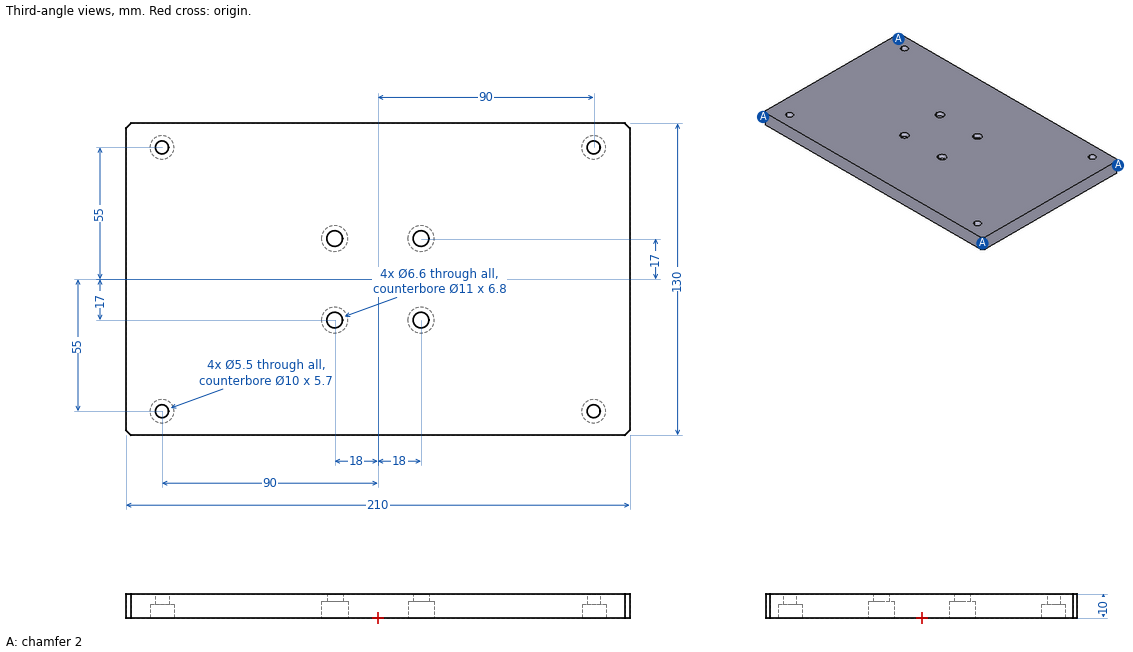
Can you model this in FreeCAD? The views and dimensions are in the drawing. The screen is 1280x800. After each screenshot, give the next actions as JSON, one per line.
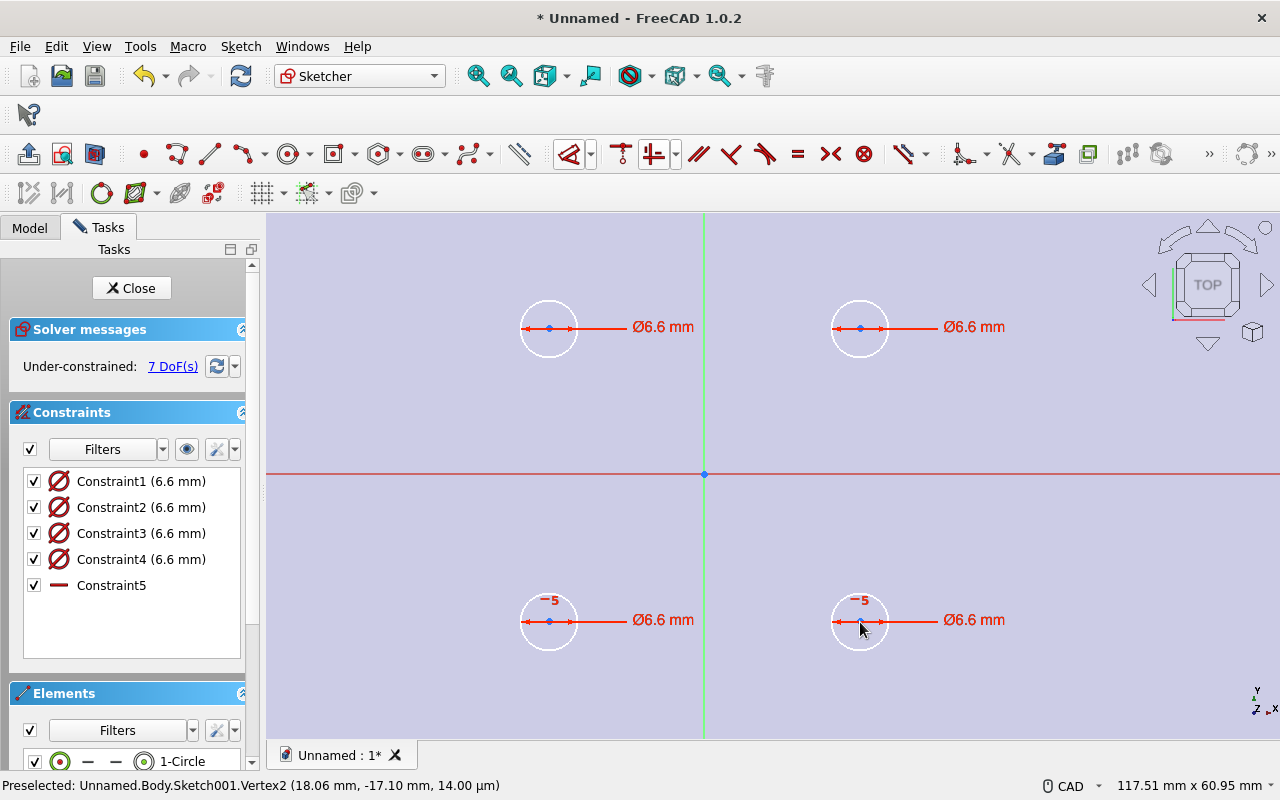
{"action": "left_click", "coordinate": [860, 622]}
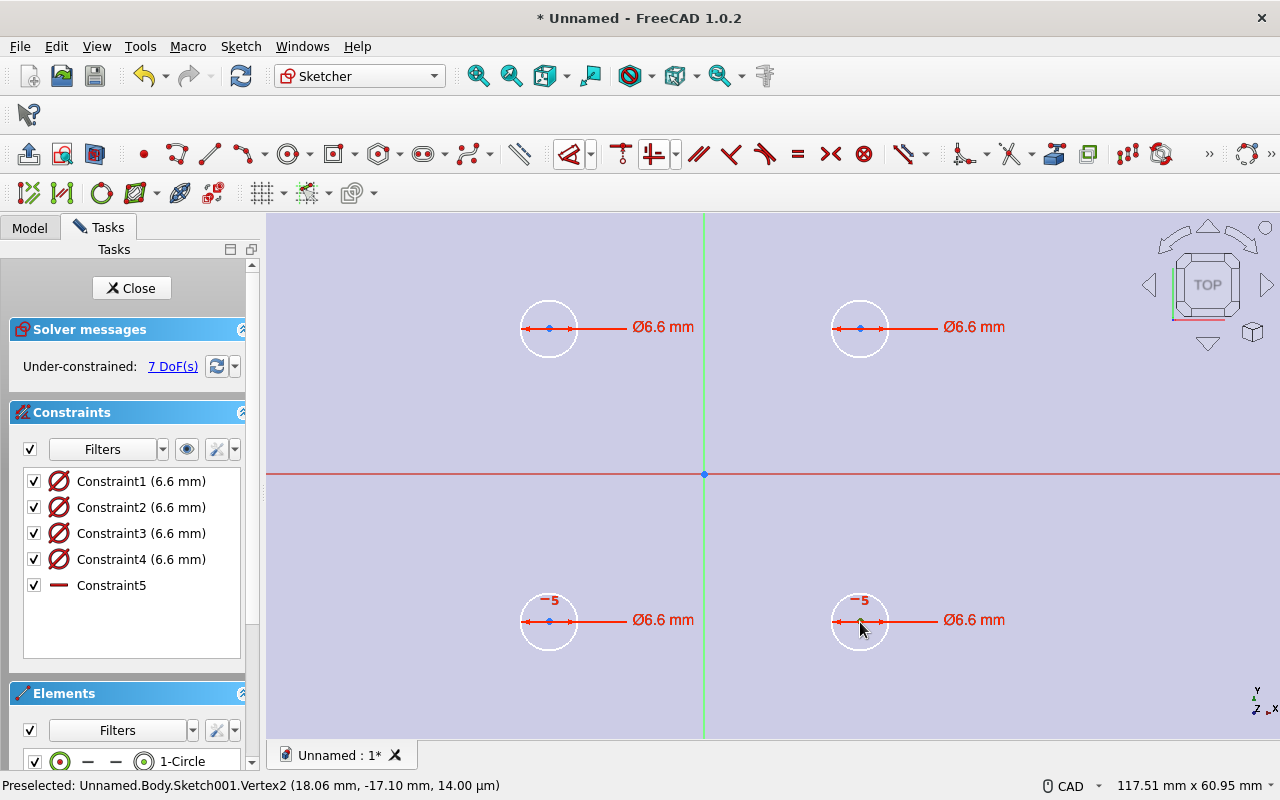
{"action": "left_click", "coordinate": [860, 329]}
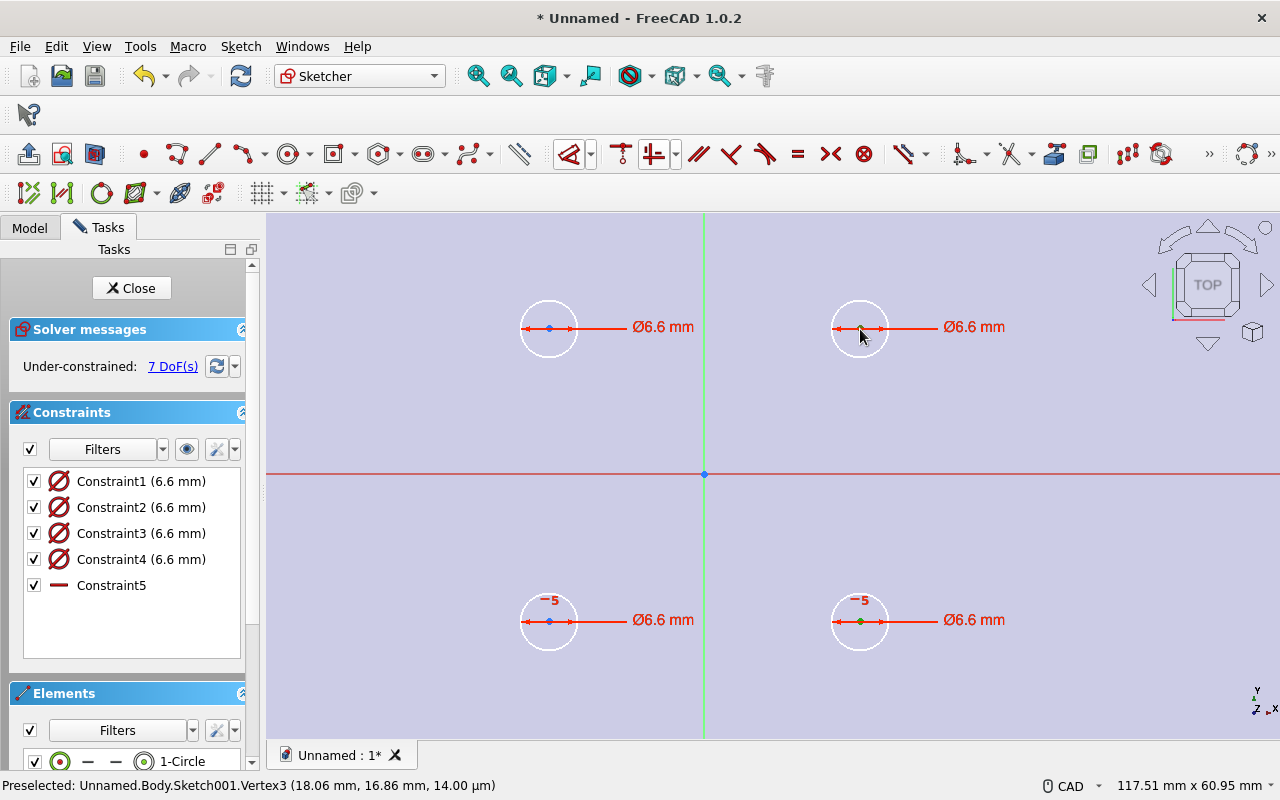
{"action": "left_click", "coordinate": [676, 154]}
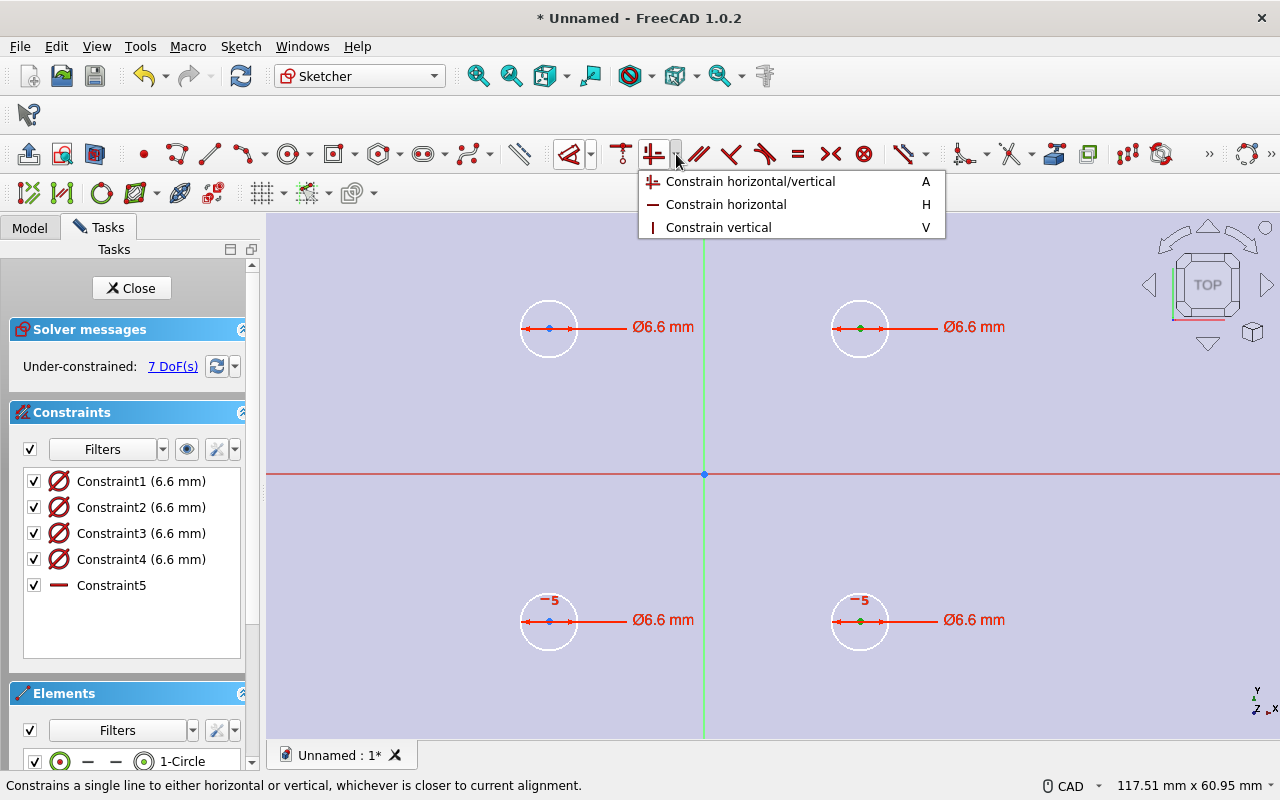
{"action": "left_click", "coordinate": [792, 228]}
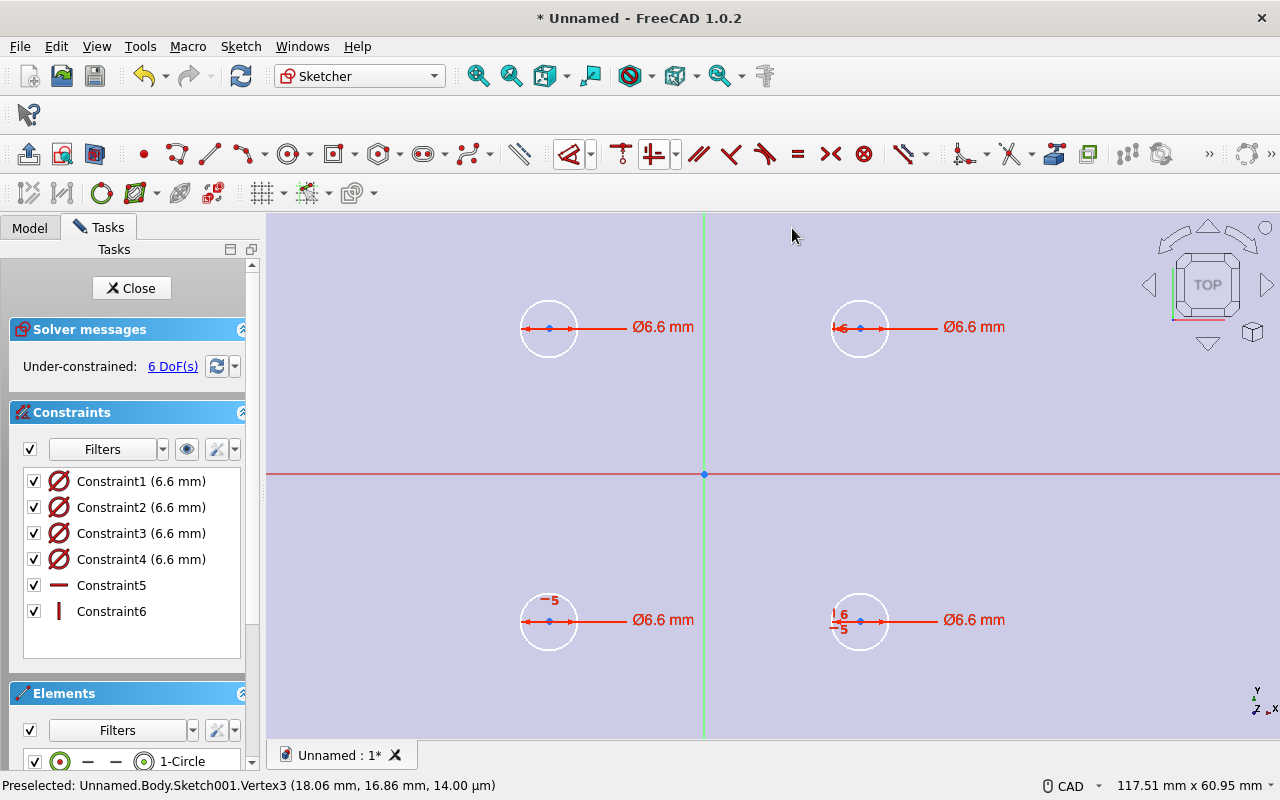
{"action": "left_click", "coordinate": [549, 622]}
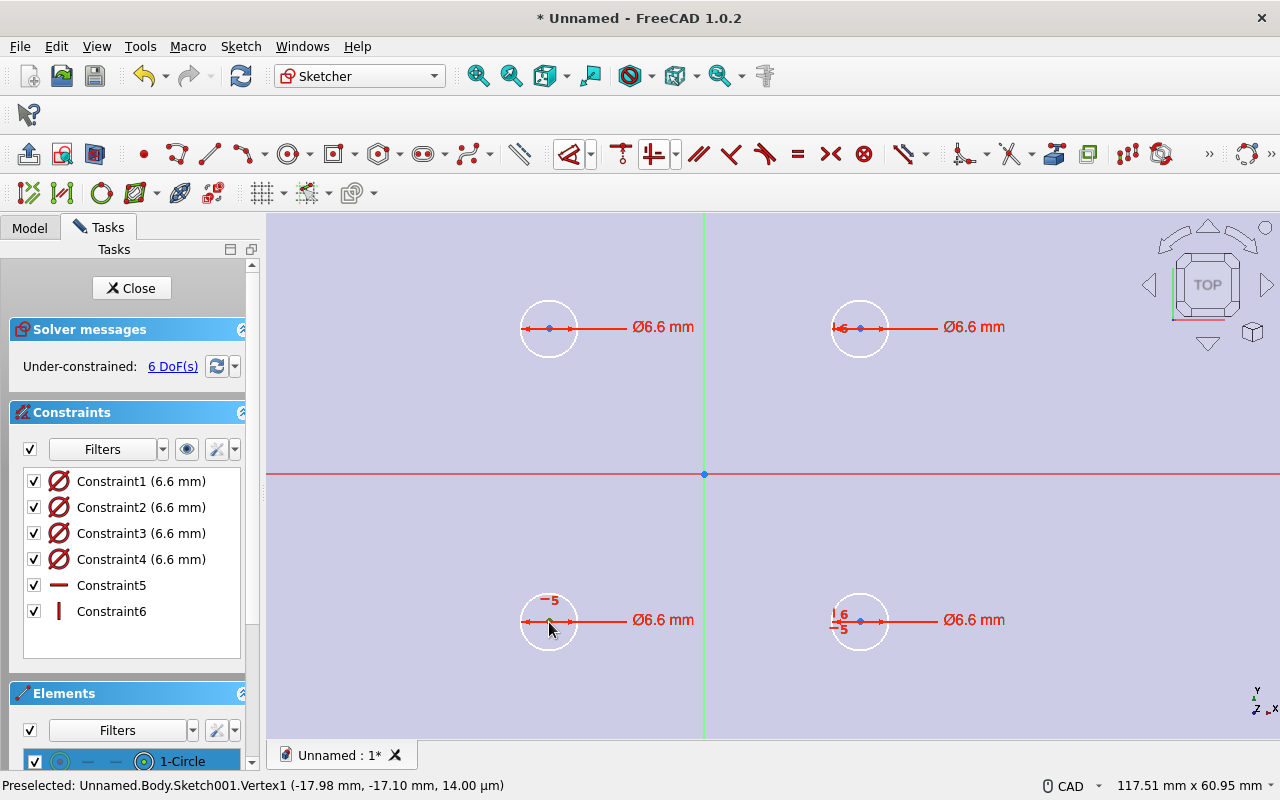
{"action": "left_click", "coordinate": [549, 329]}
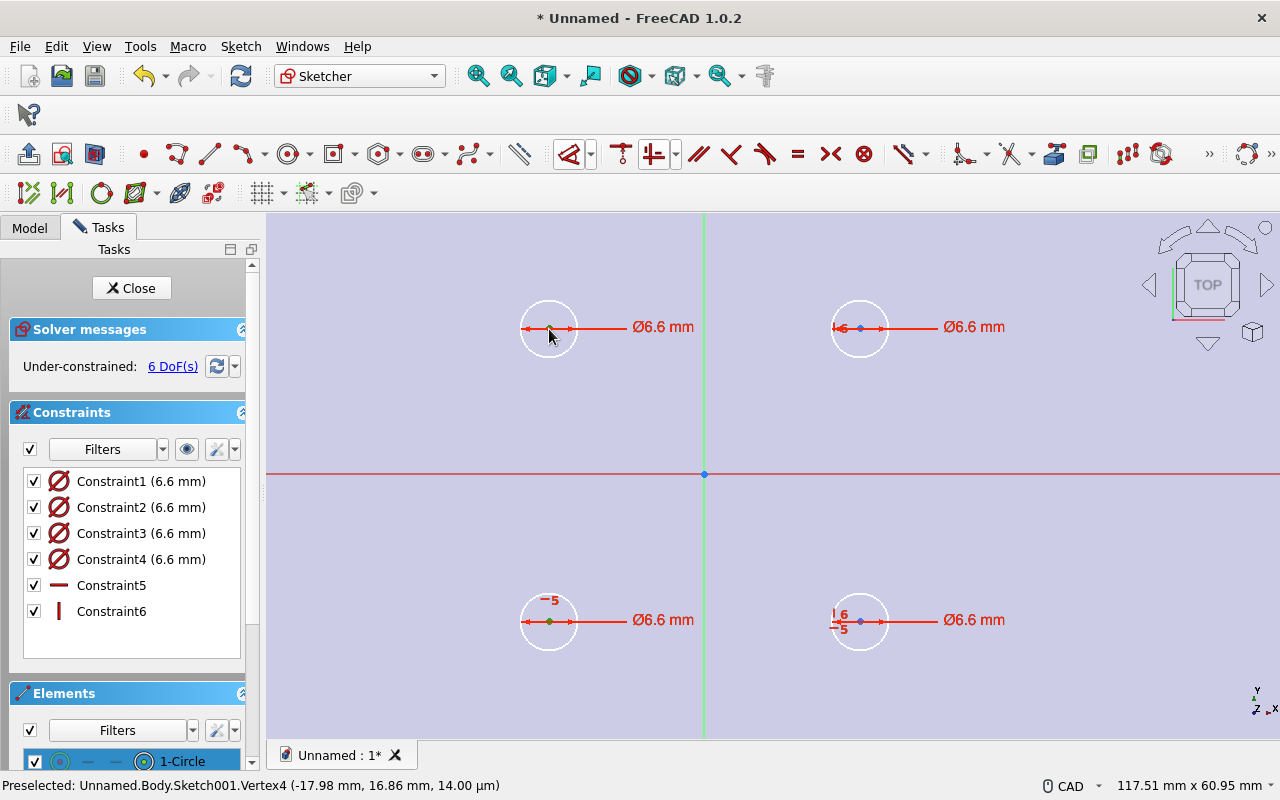
{"action": "left_click", "coordinate": [676, 154]}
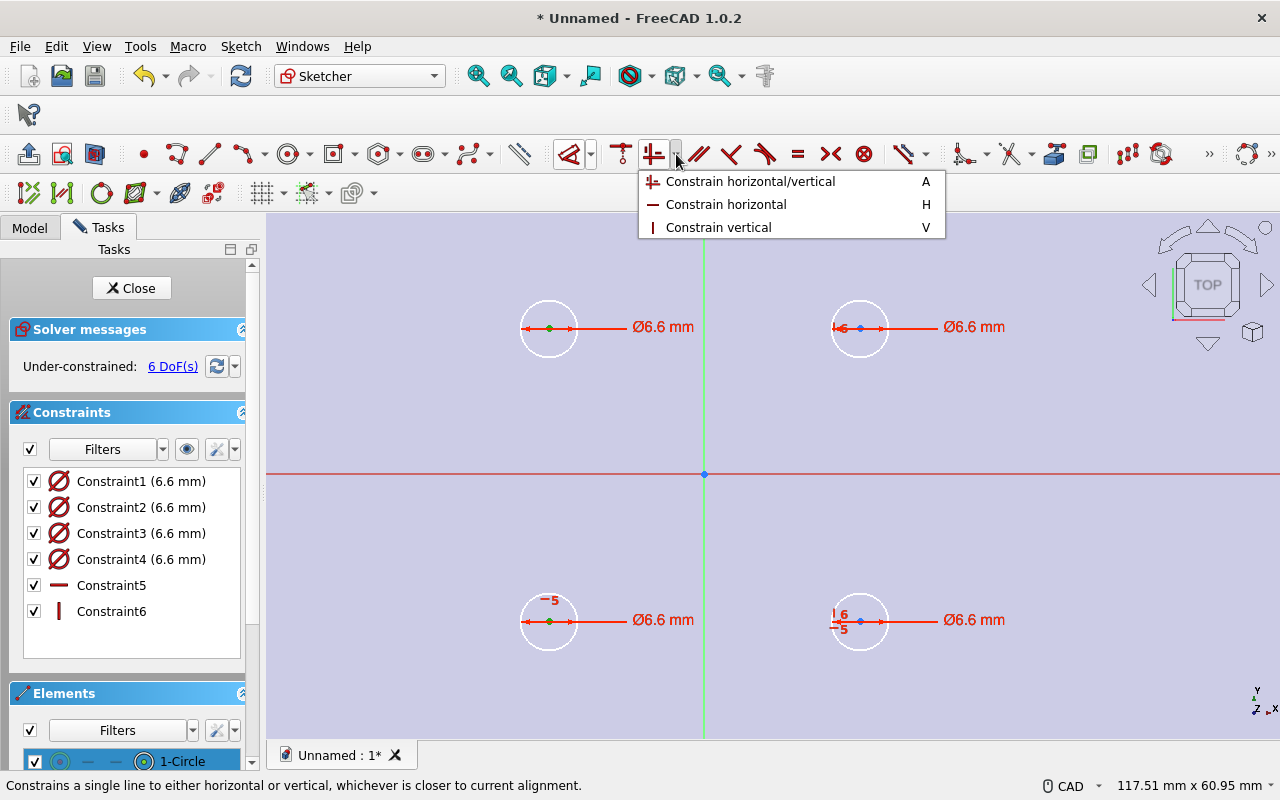
{"action": "left_click", "coordinate": [792, 228]}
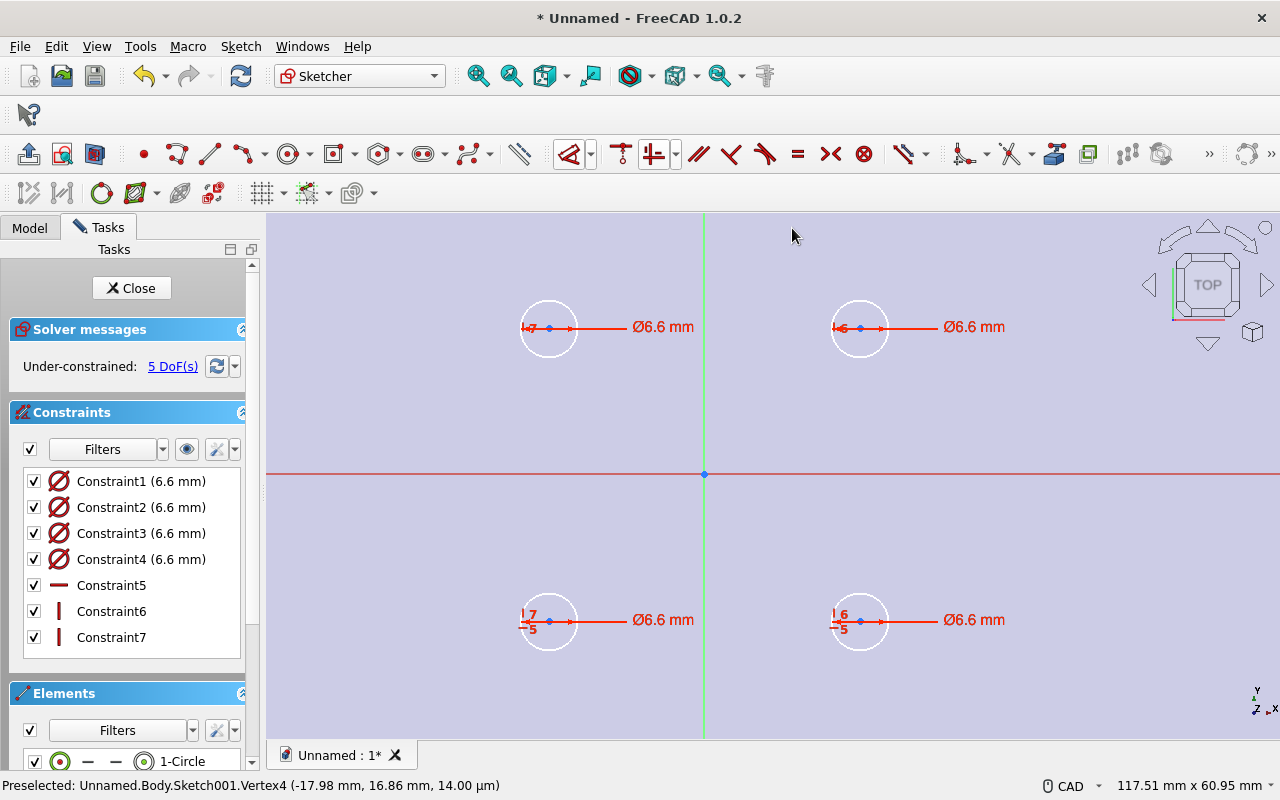
{"action": "left_click", "coordinate": [860, 329]}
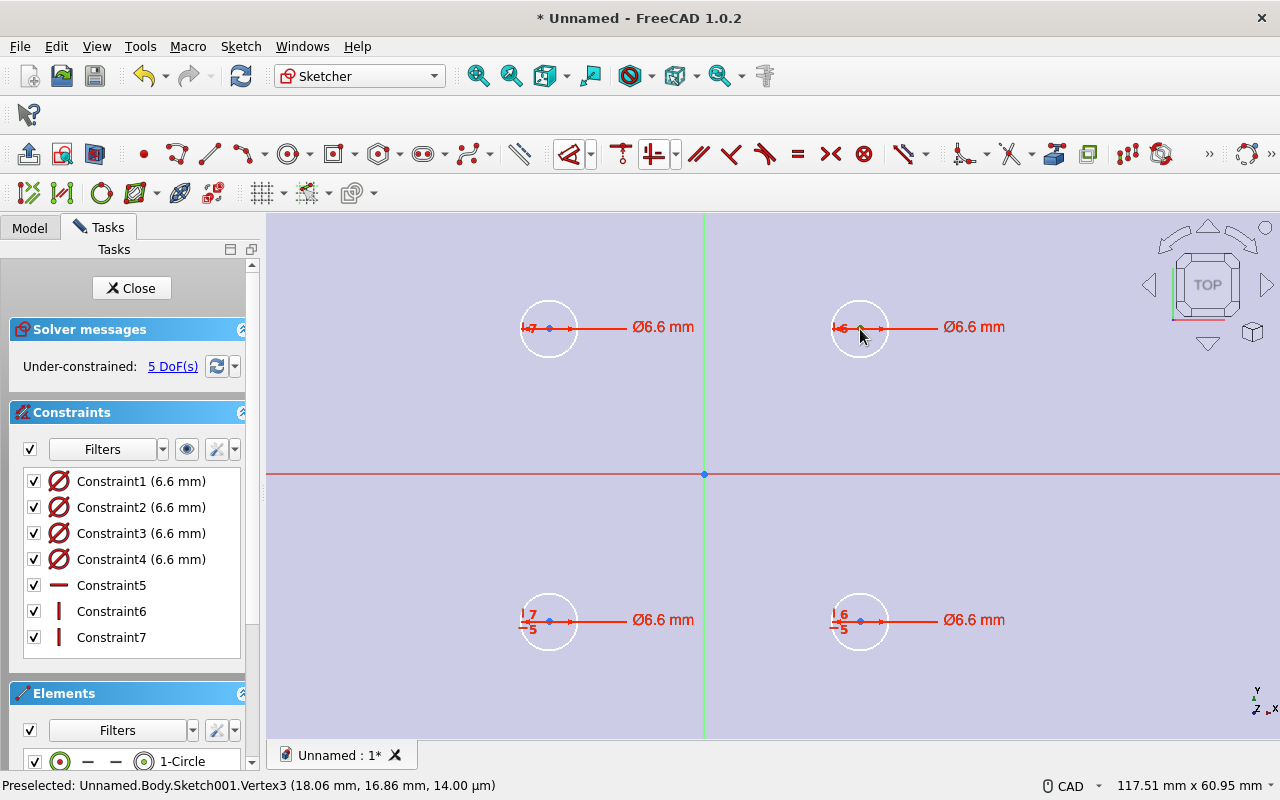
{"action": "left_click", "coordinate": [549, 329]}